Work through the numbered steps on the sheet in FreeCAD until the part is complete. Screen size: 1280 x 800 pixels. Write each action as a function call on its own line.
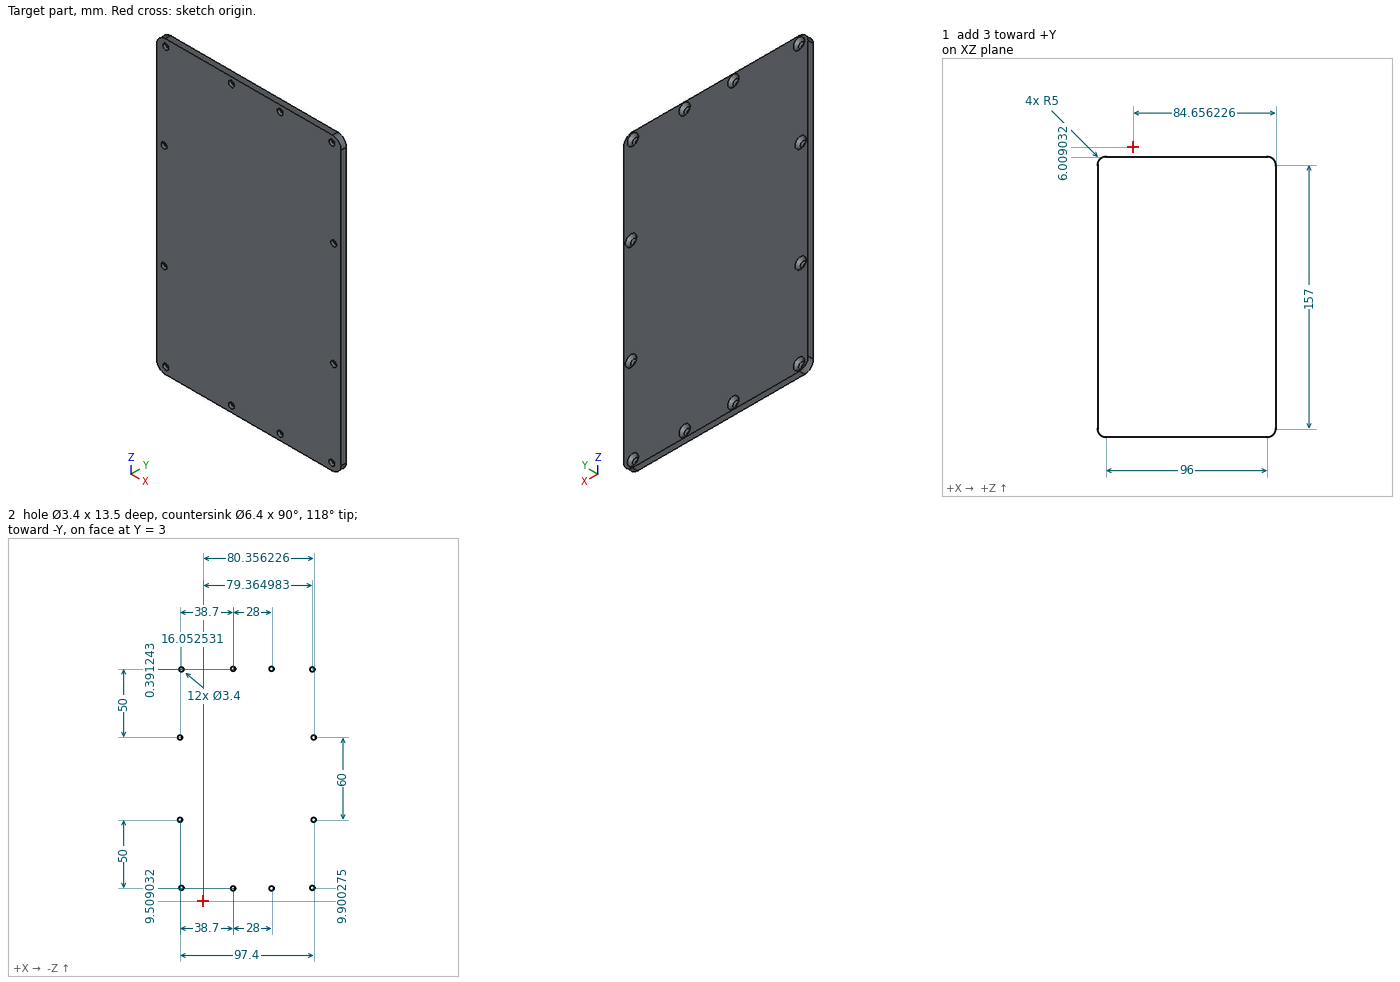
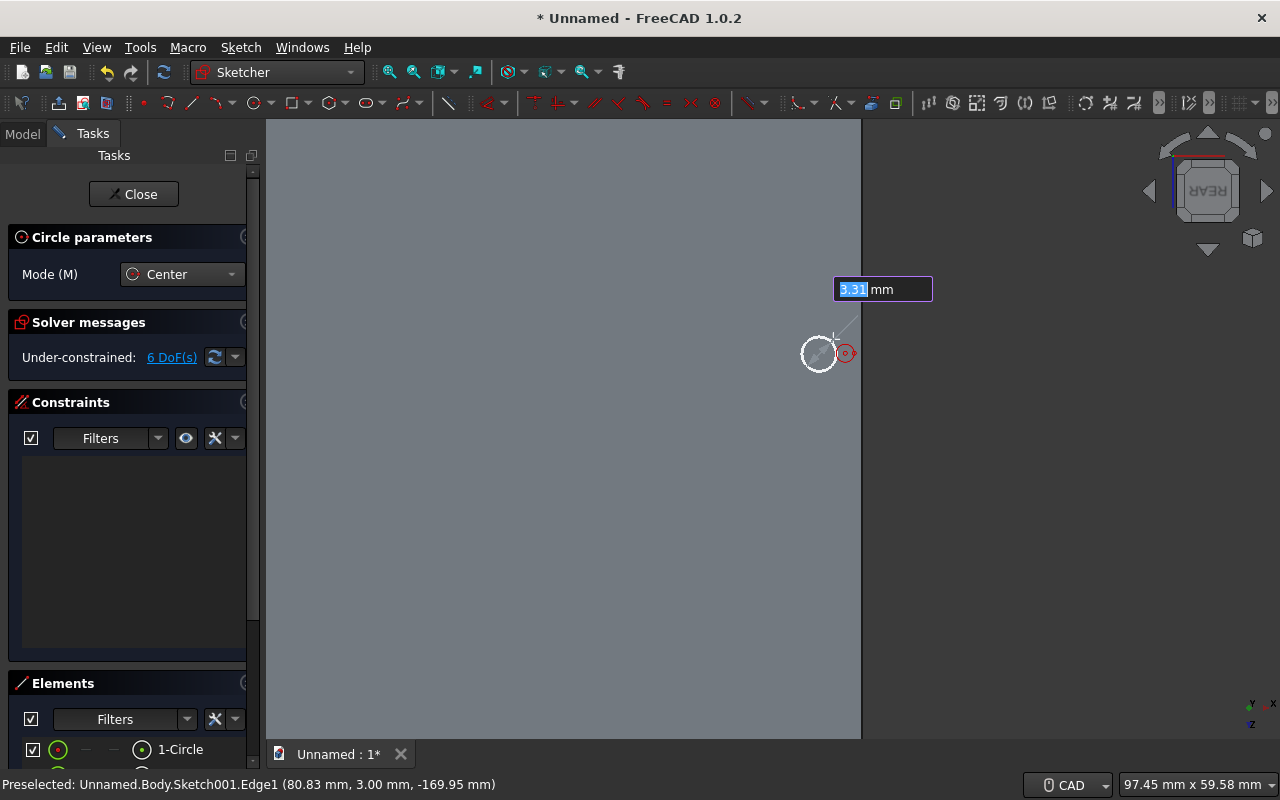
click(830, 338)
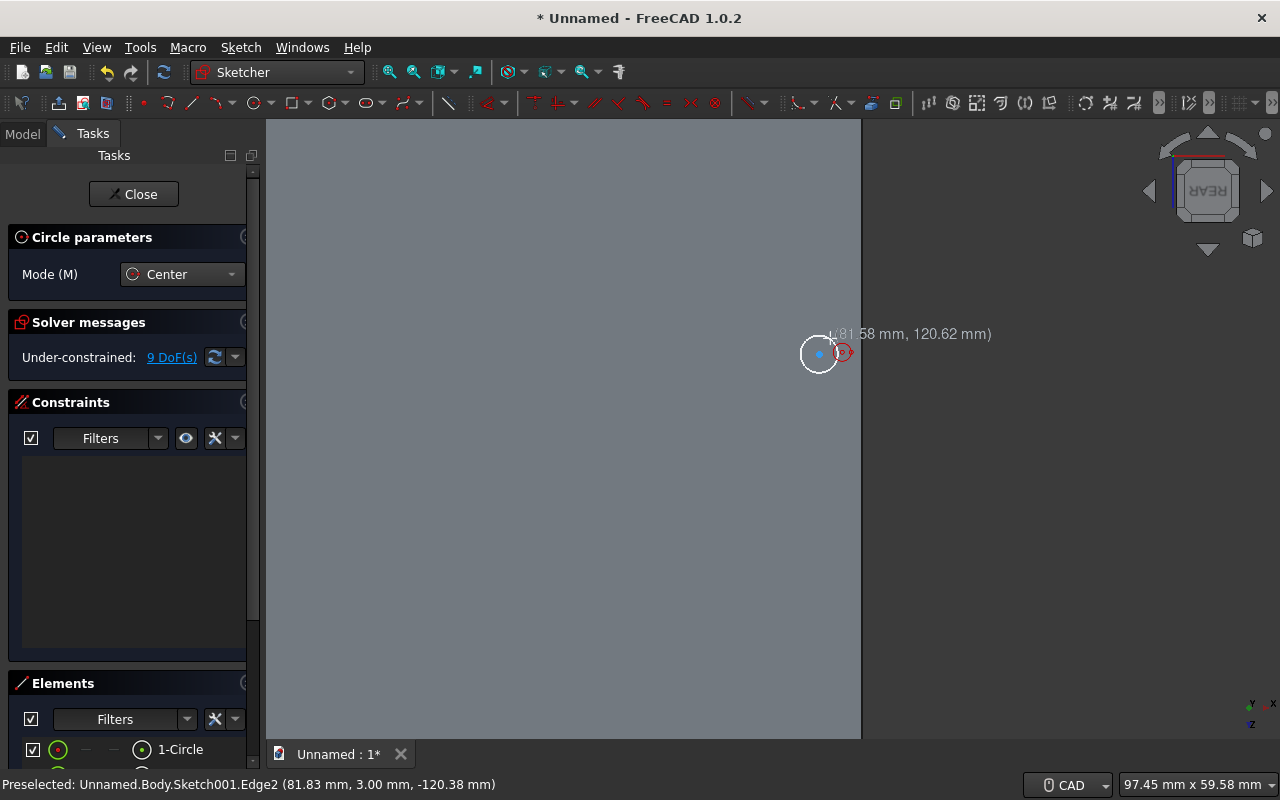
scroll(833, 339, down, 7)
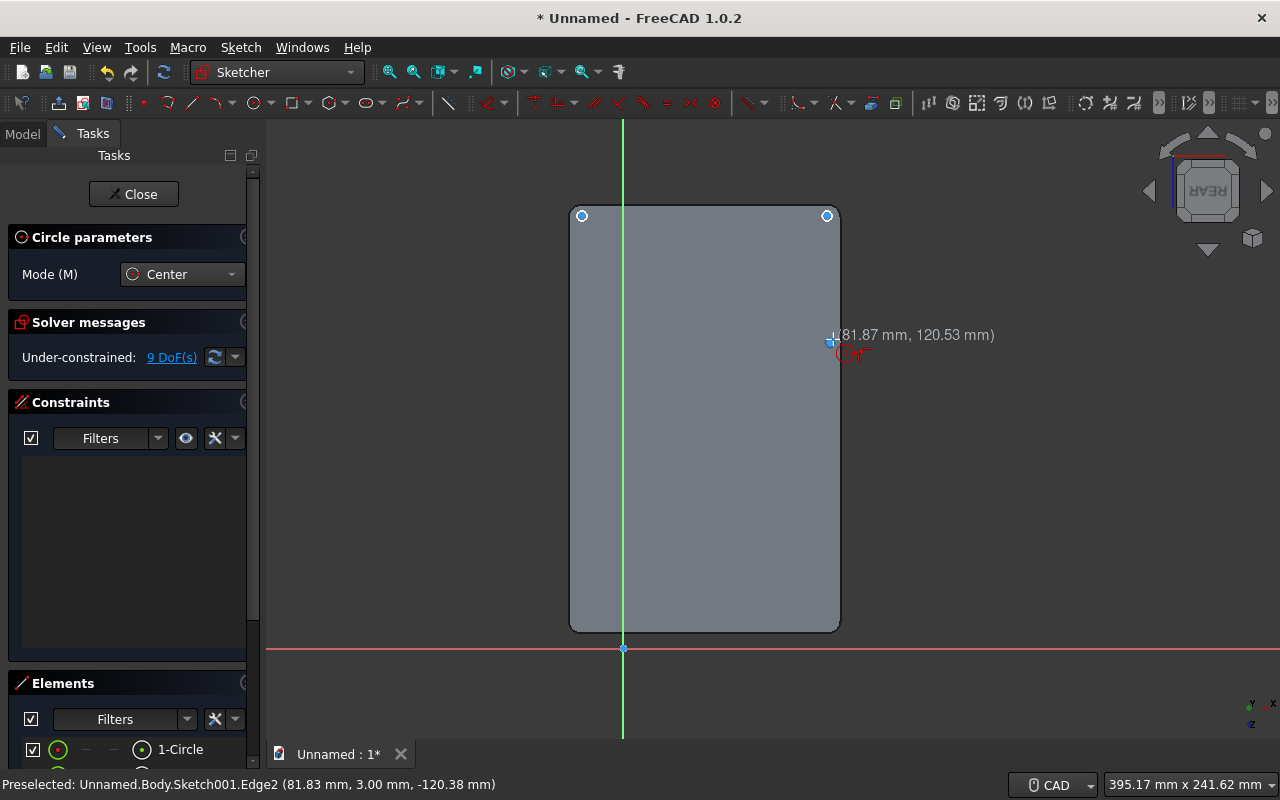
scroll(830, 496, up, 9)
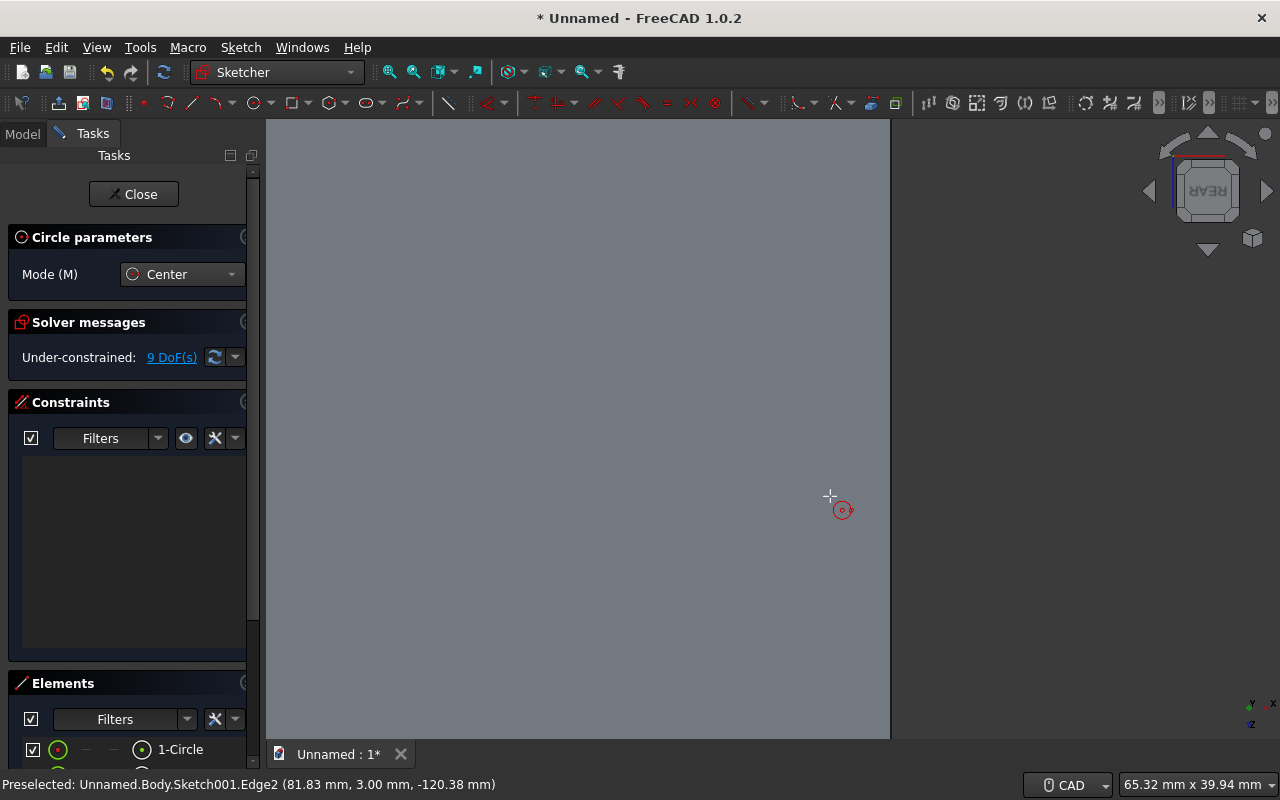
scroll(830, 496, down, 9)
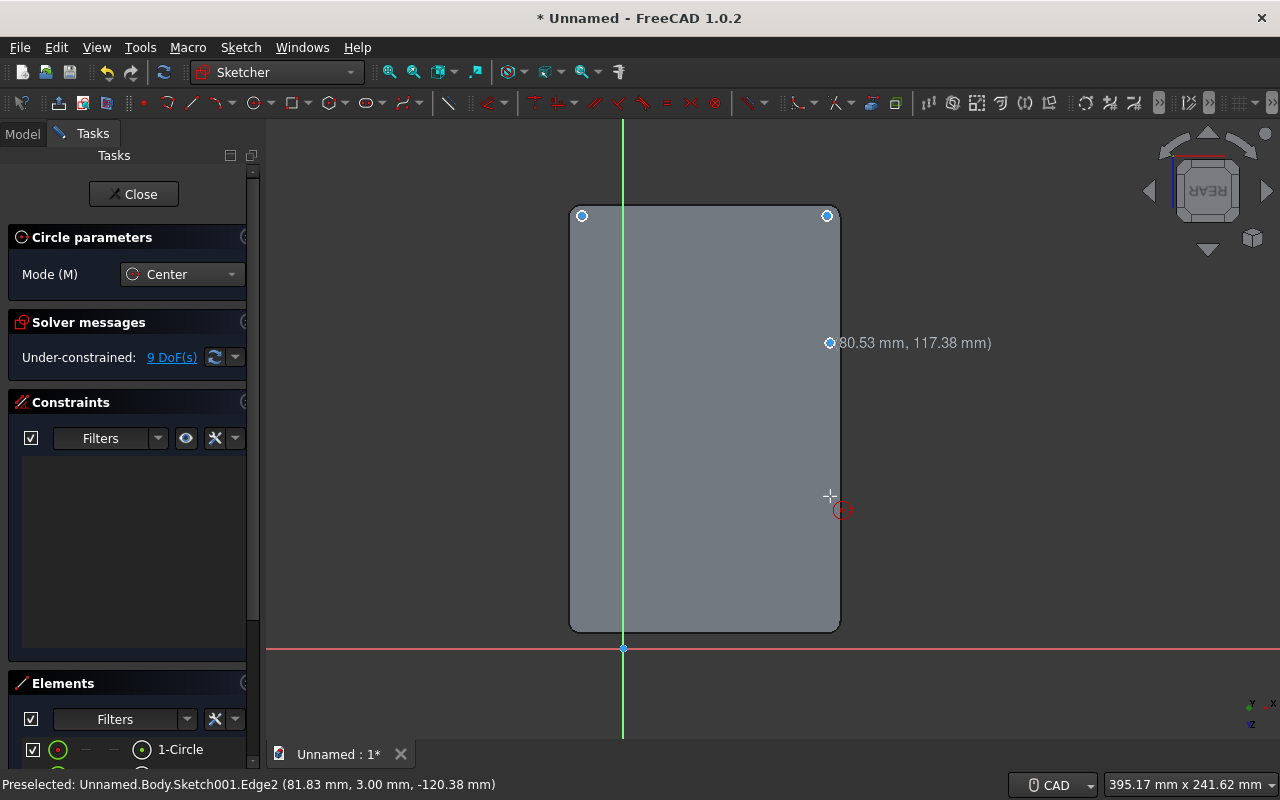
click(830, 496)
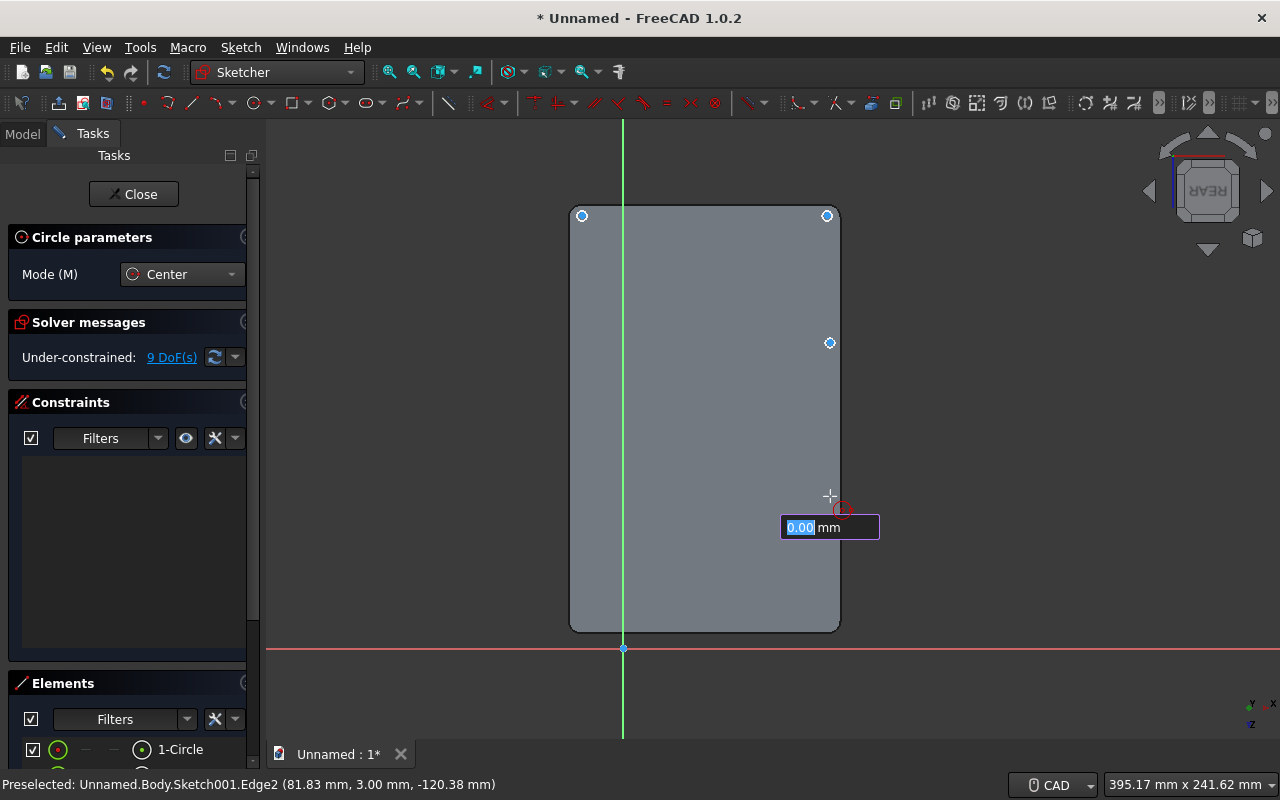
scroll(833, 493, up, 7)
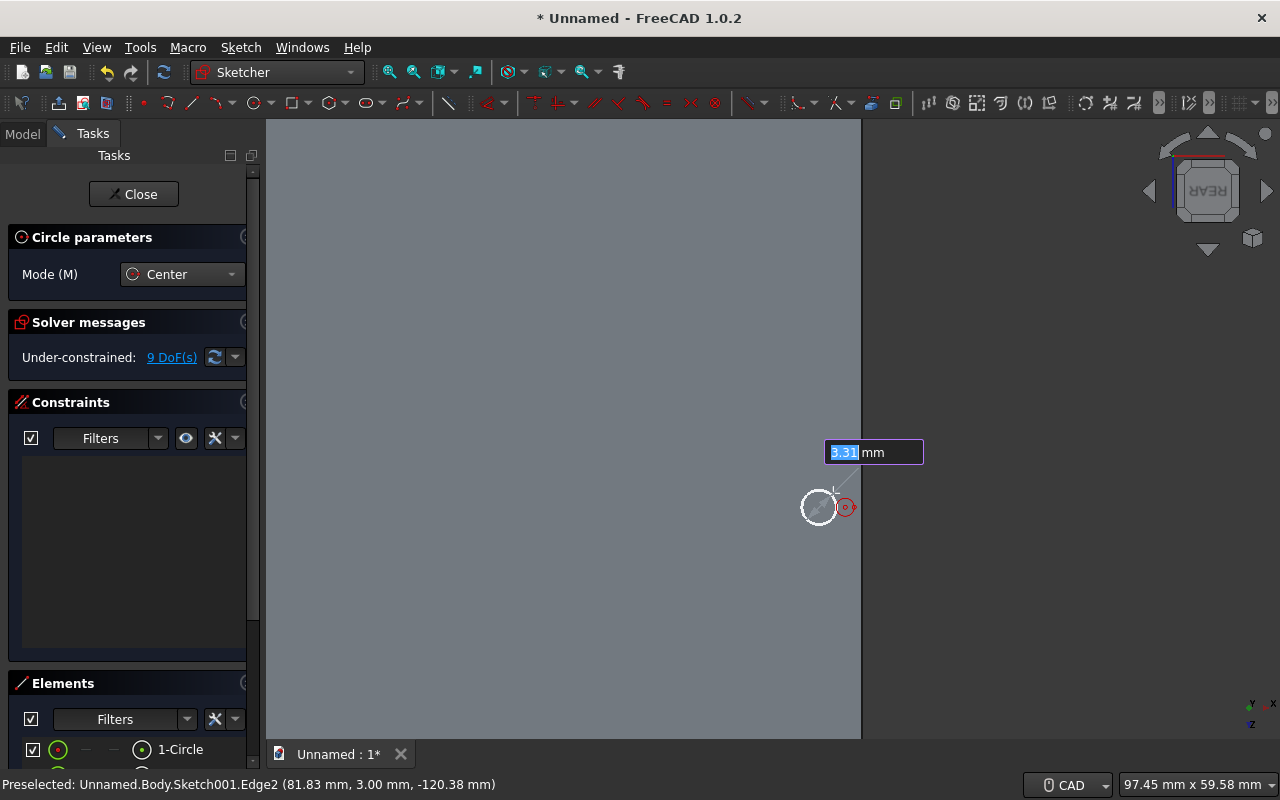
click(830, 491)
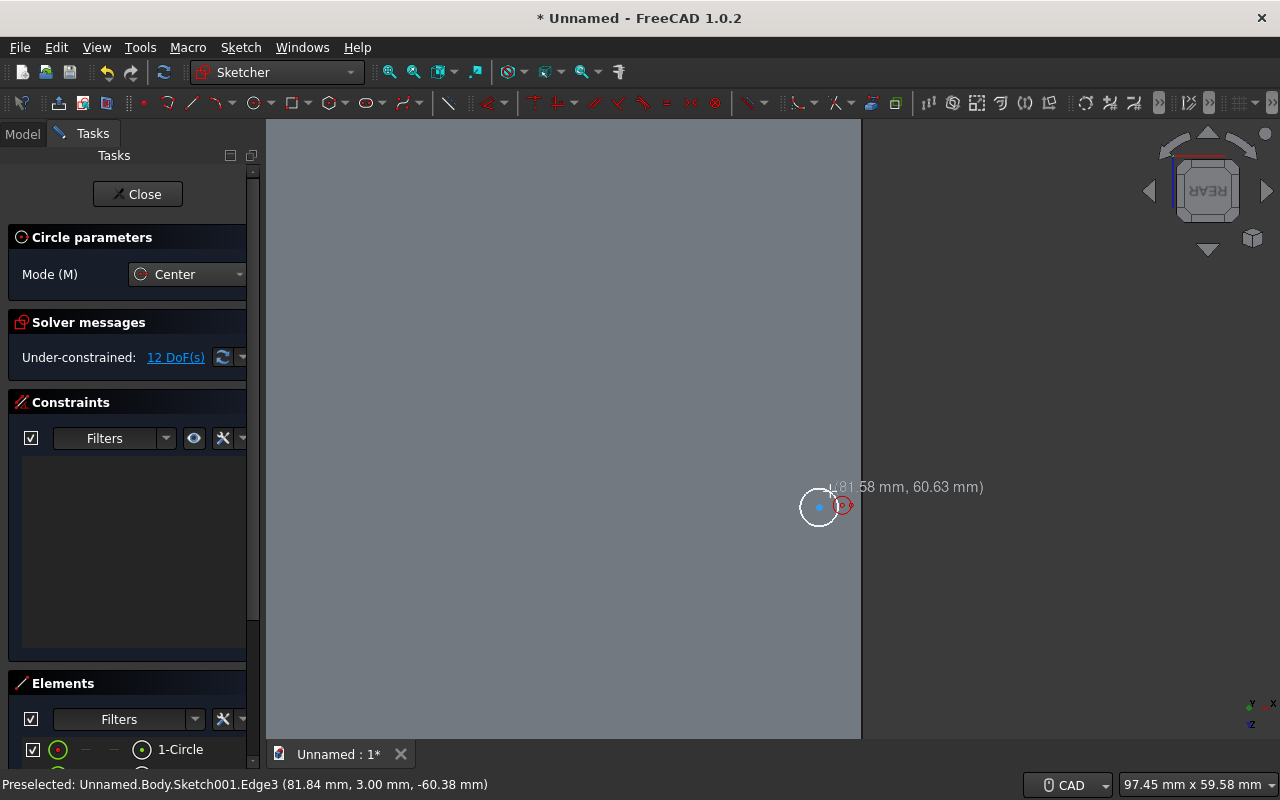
scroll(833, 493, down, 7)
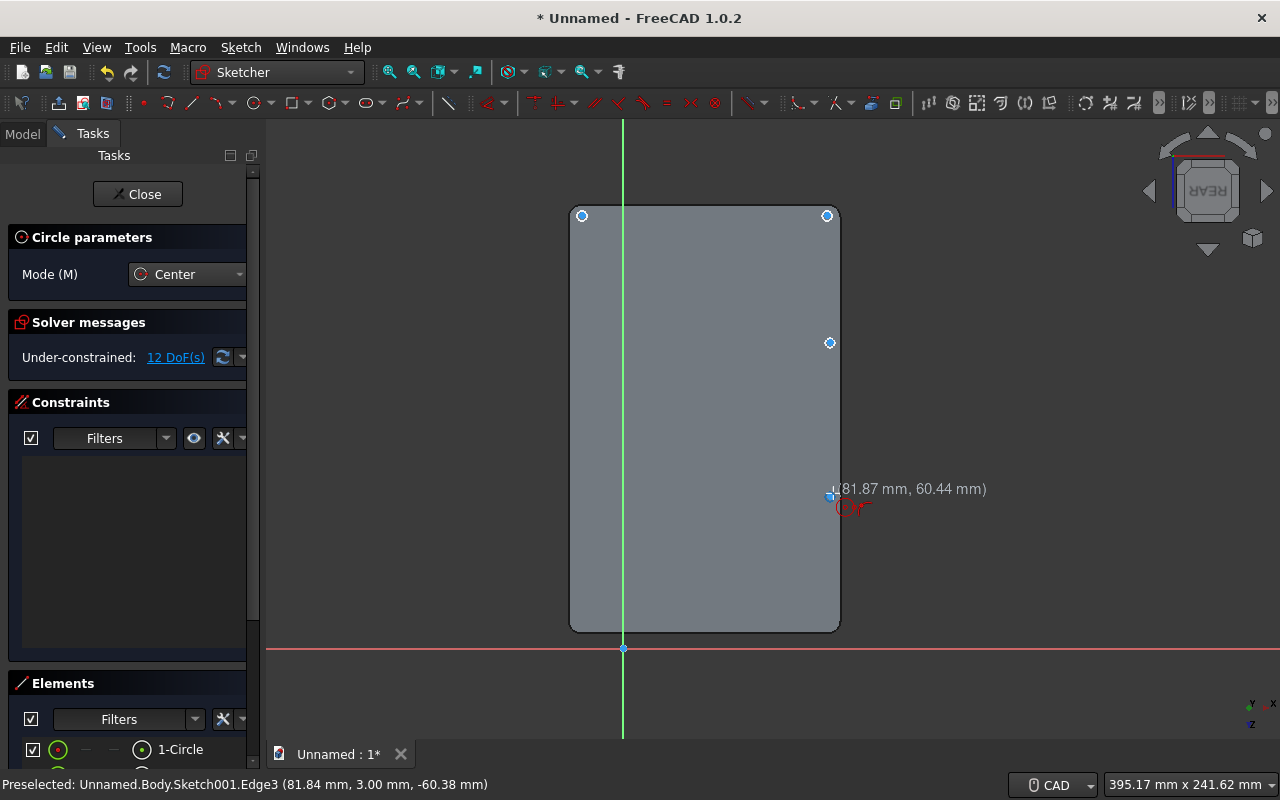
scroll(827, 623, up, 9)